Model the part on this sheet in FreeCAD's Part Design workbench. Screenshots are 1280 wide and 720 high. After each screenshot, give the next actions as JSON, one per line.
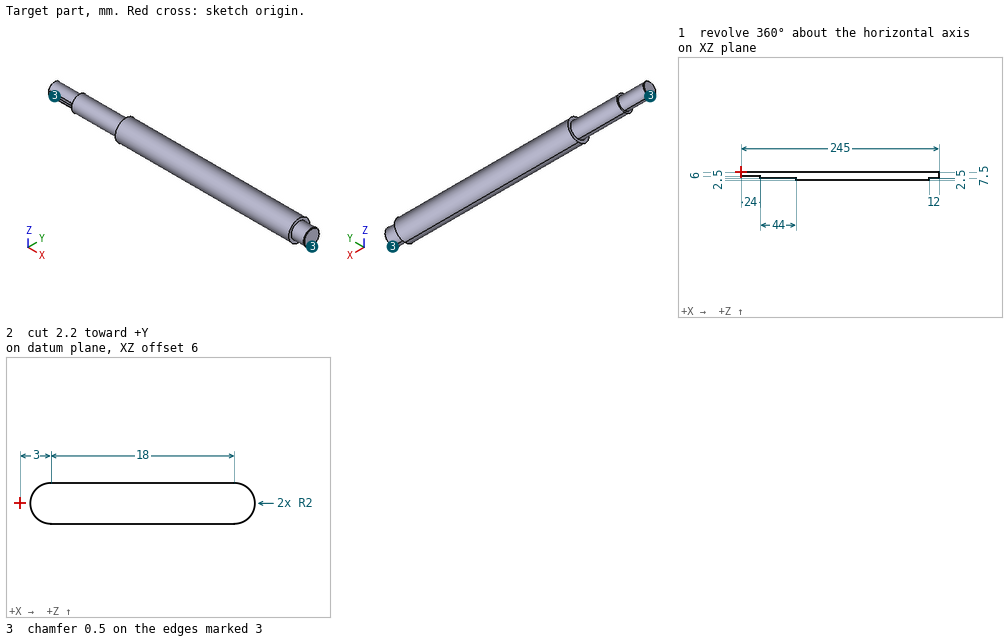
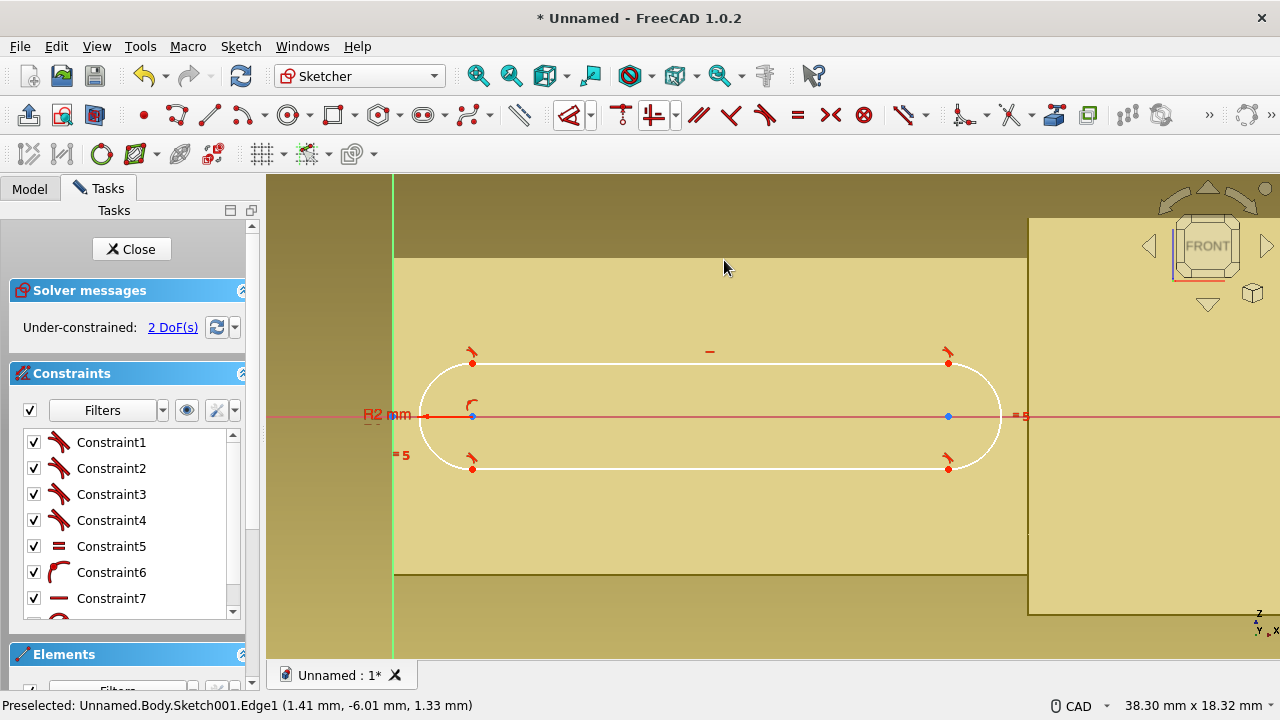
{"action": "left_click", "coordinate": [615, 364]}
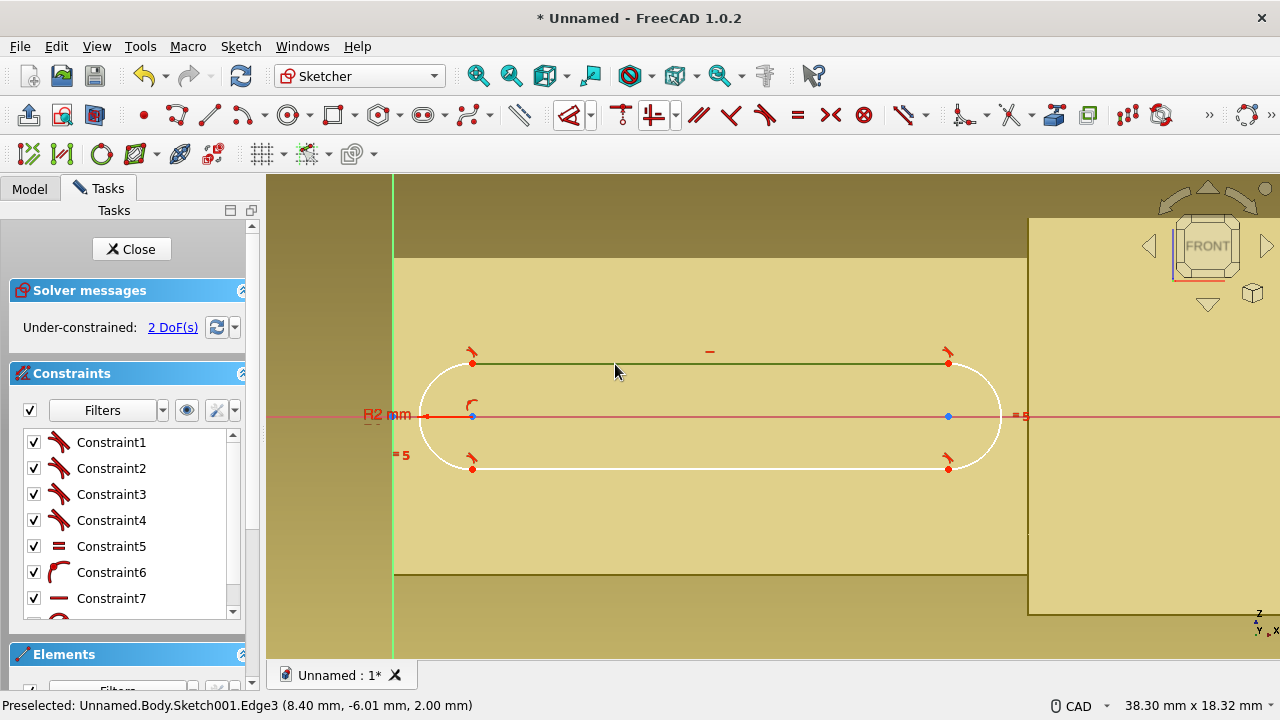
{"action": "left_click", "coordinate": [590, 116]}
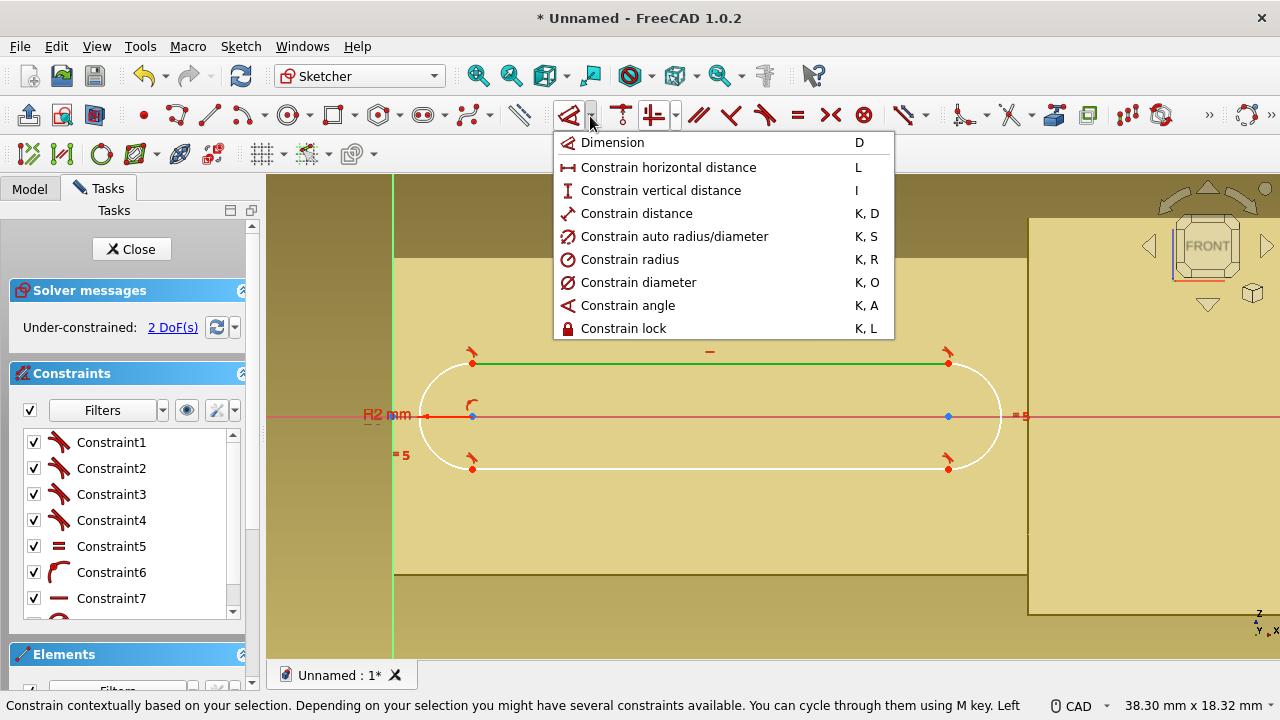
{"action": "left_click", "coordinate": [724, 168]}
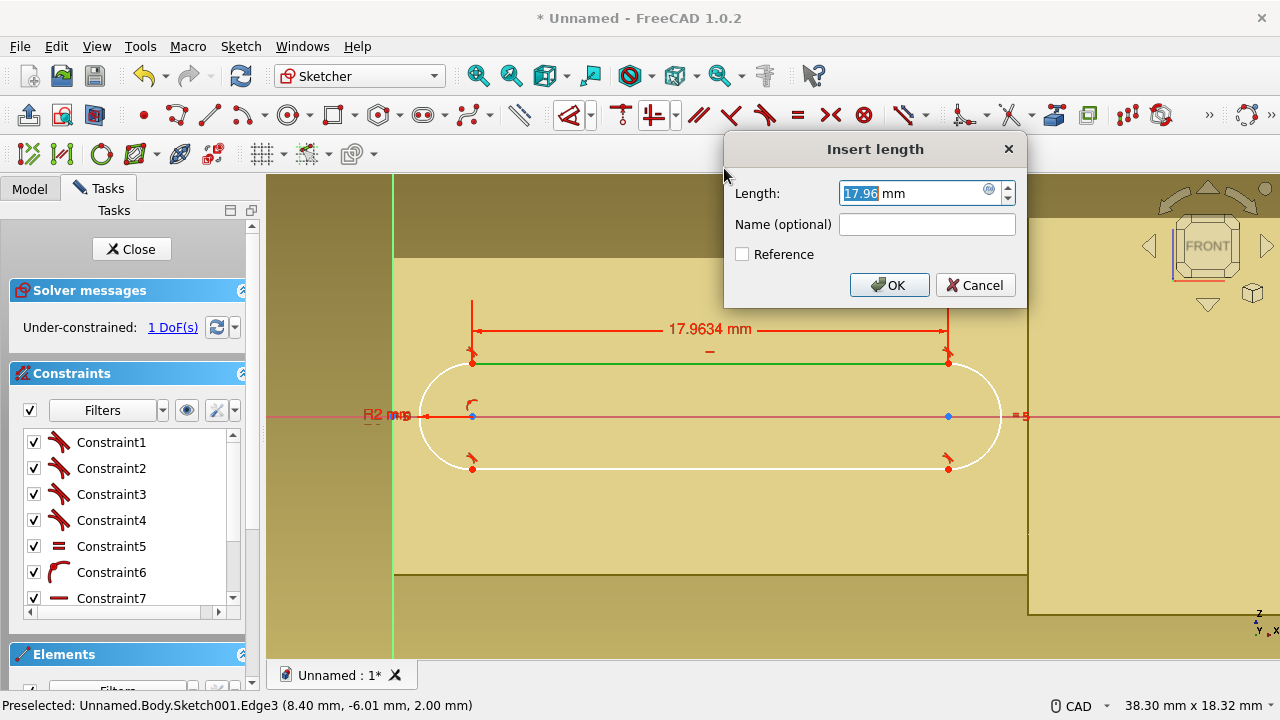
{"action": "type", "text": "18"}
{"action": "key", "text": "Return"}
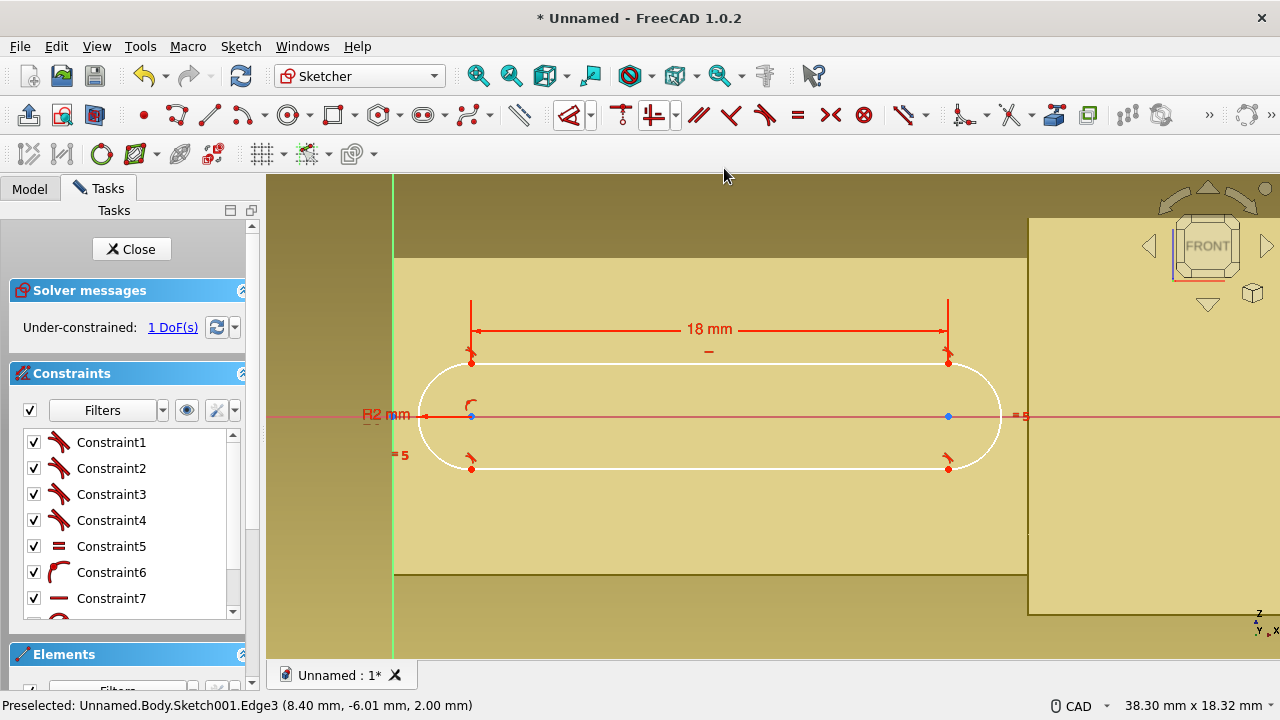
{"action": "left_click", "coordinate": [471, 364]}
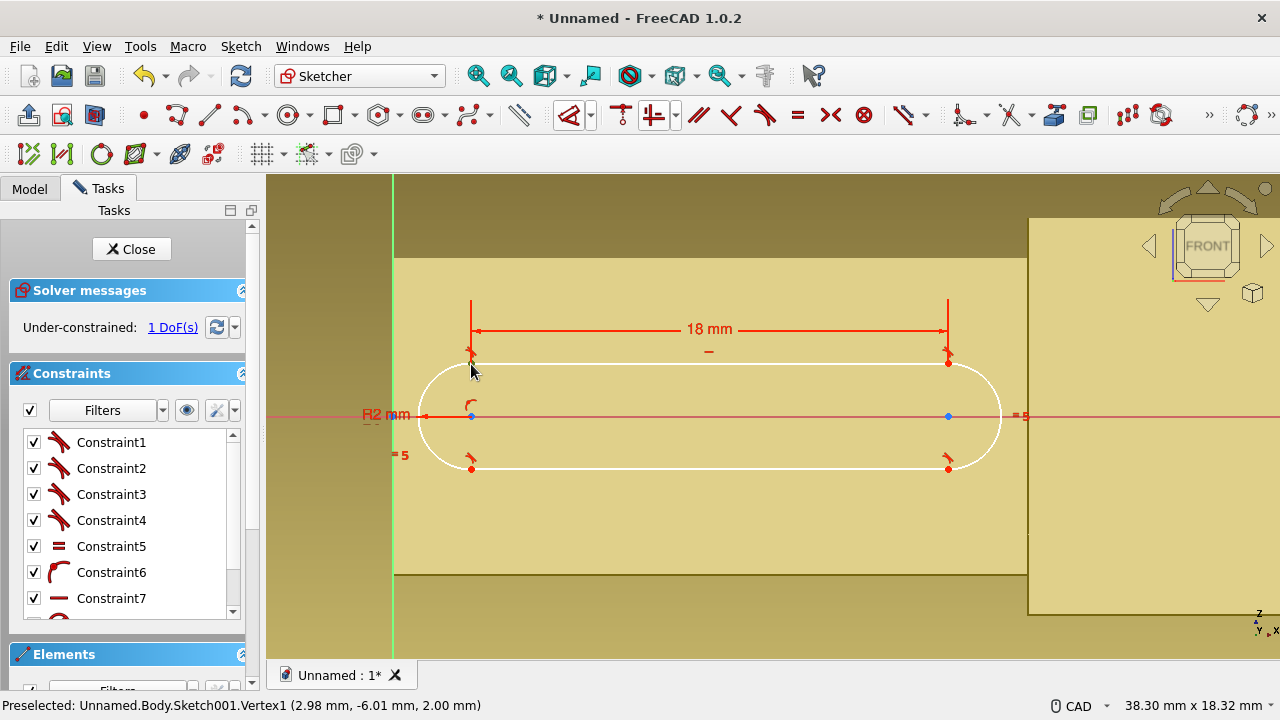
{"action": "key", "text": "l"}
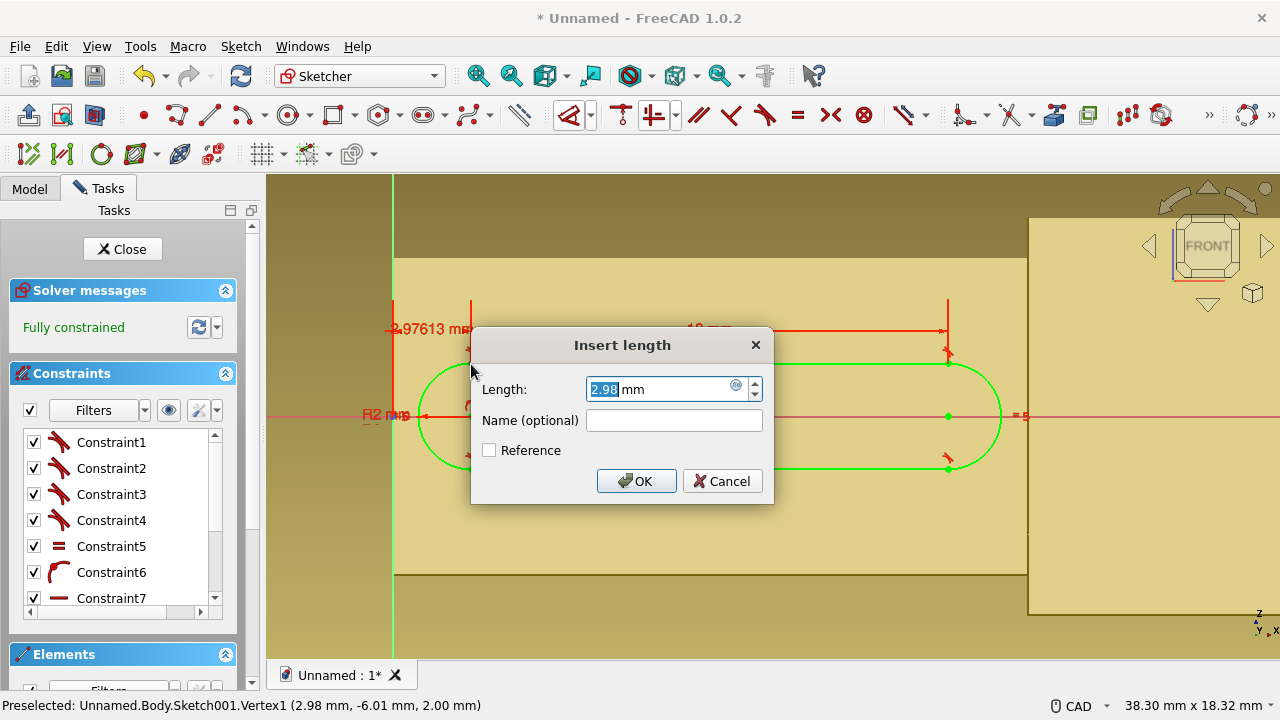
{"action": "type", "text": "3"}
{"action": "key", "text": "Return"}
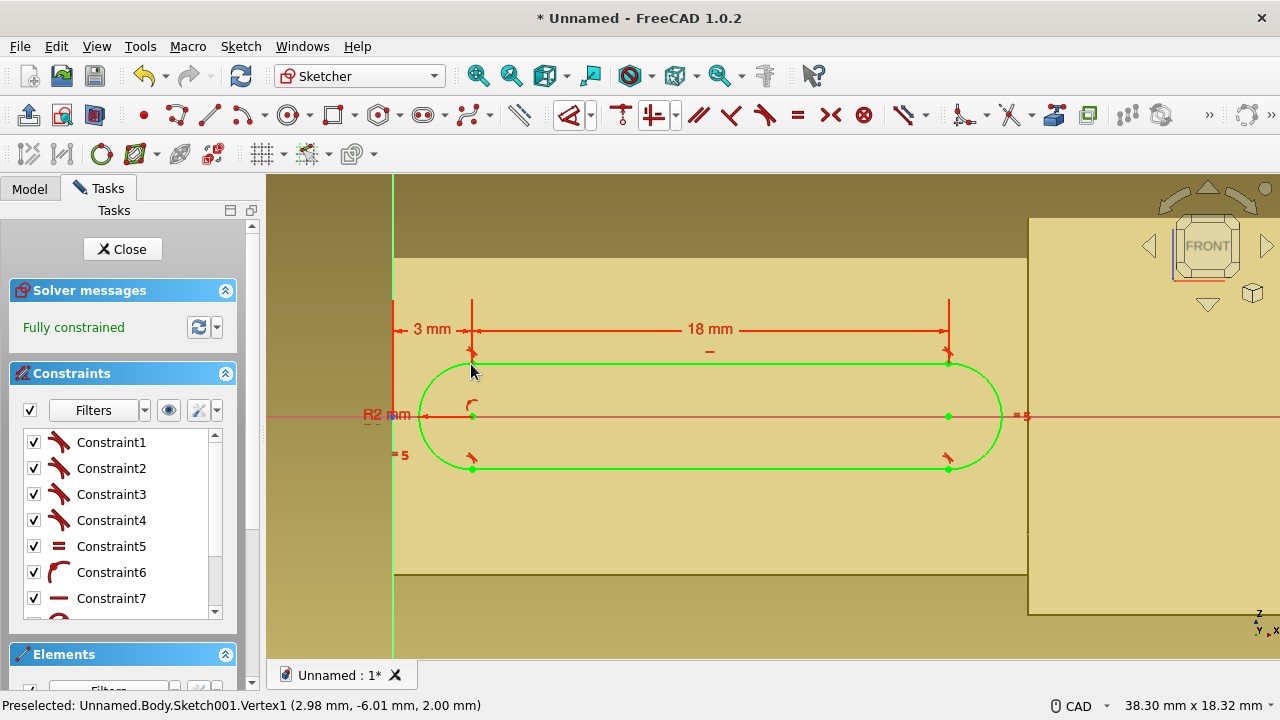
{"action": "left_click", "coordinate": [123, 249]}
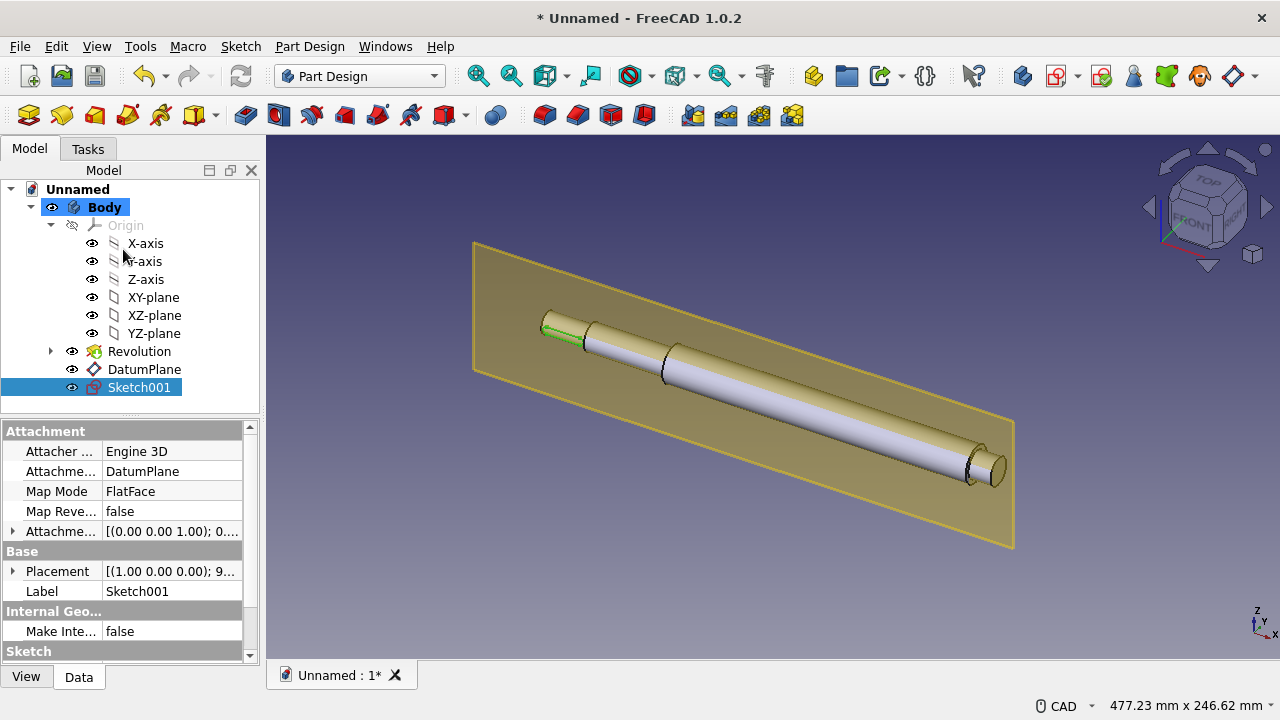
{"action": "left_click", "coordinate": [246, 116]}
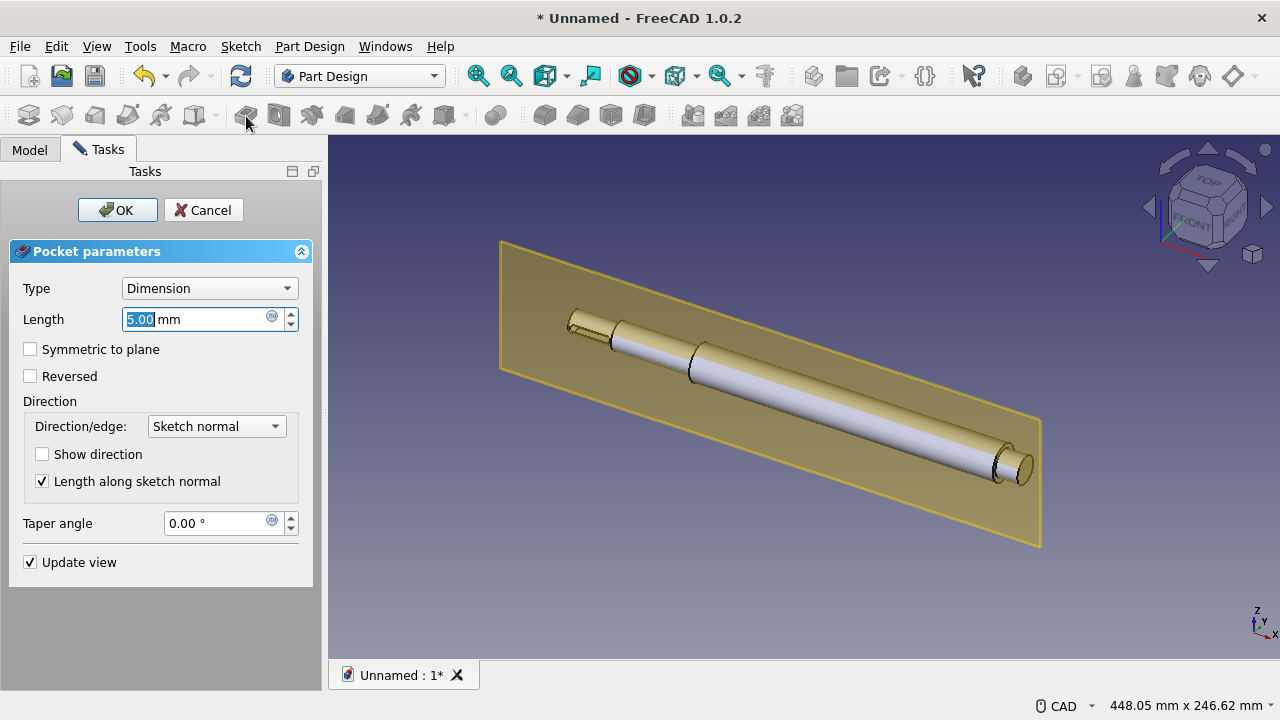
{"action": "type", "text": "2.2"}
{"action": "key", "text": "Tab"}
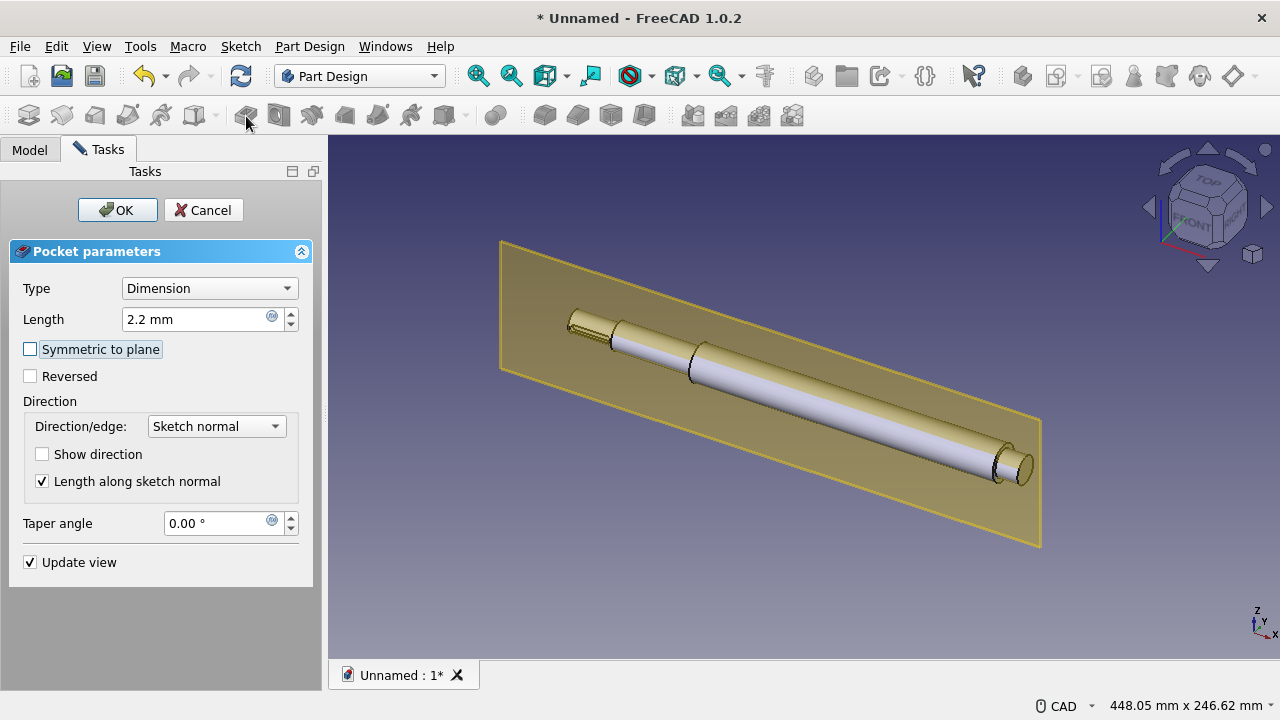
{"action": "left_click", "coordinate": [118, 210]}